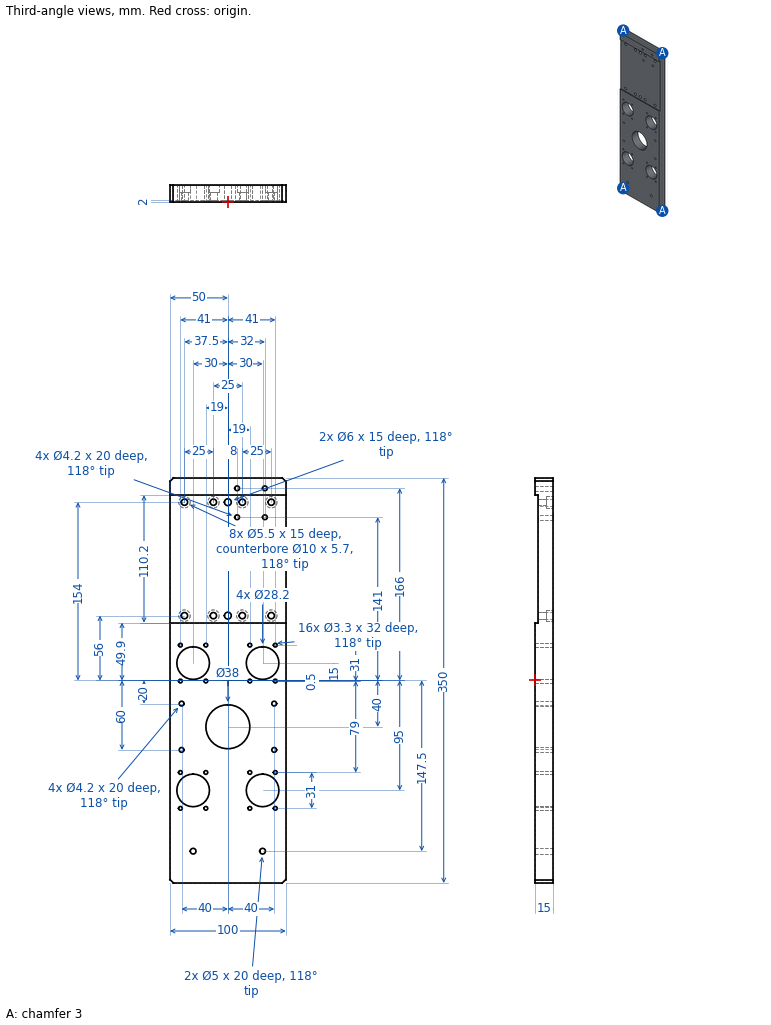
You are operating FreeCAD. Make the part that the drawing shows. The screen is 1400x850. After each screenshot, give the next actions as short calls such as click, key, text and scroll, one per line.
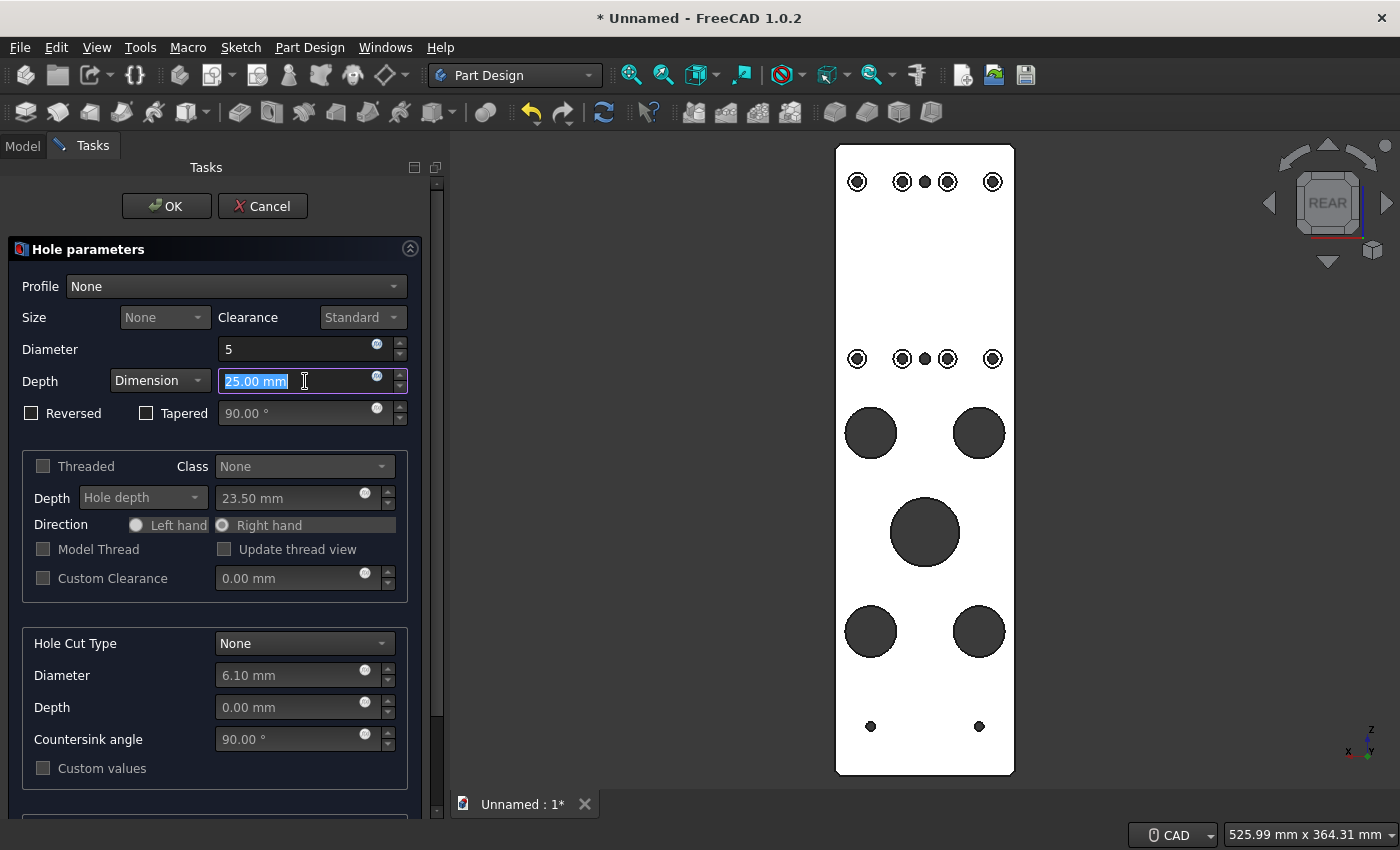
text(20)
key(Tab)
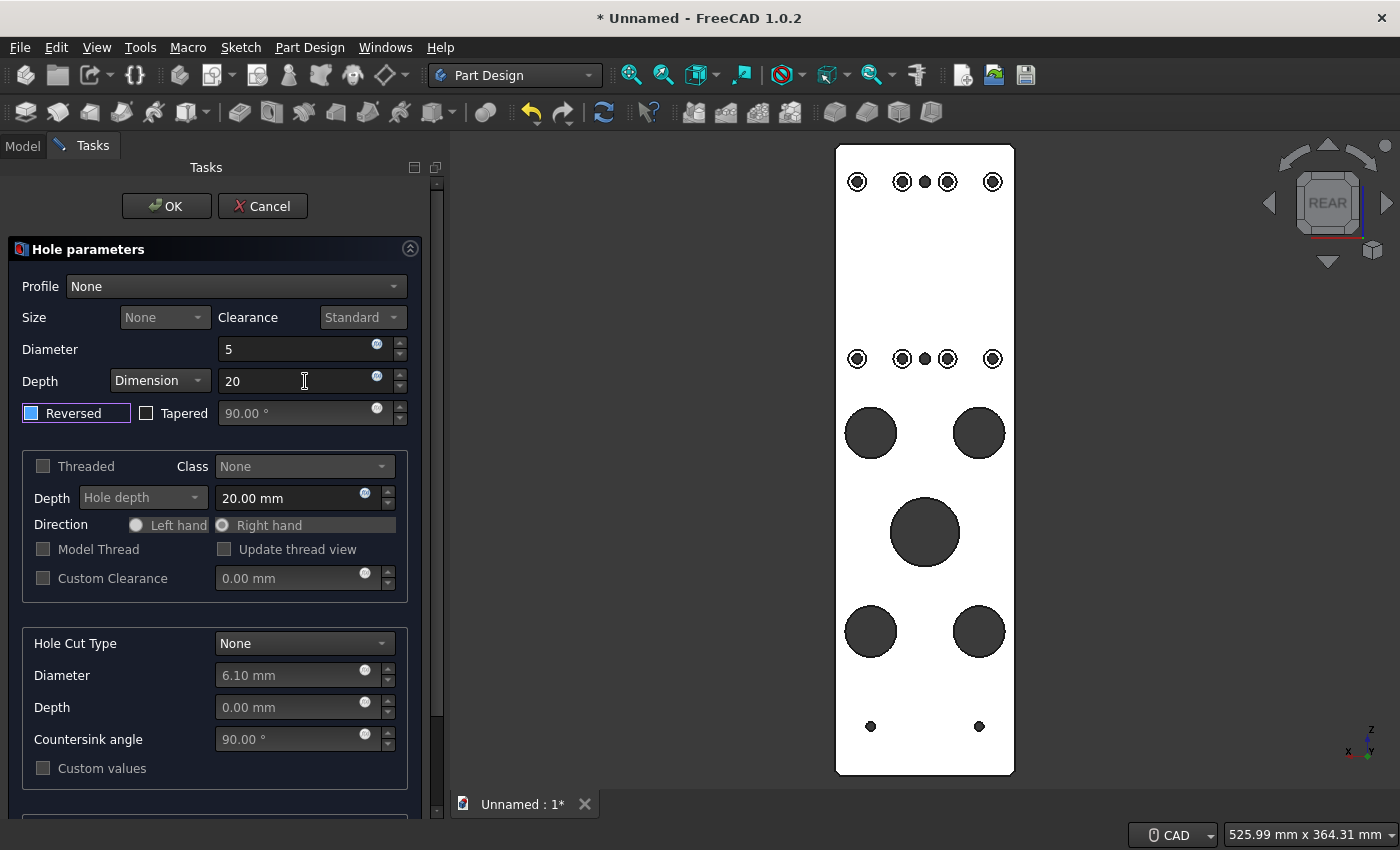
click(167, 206)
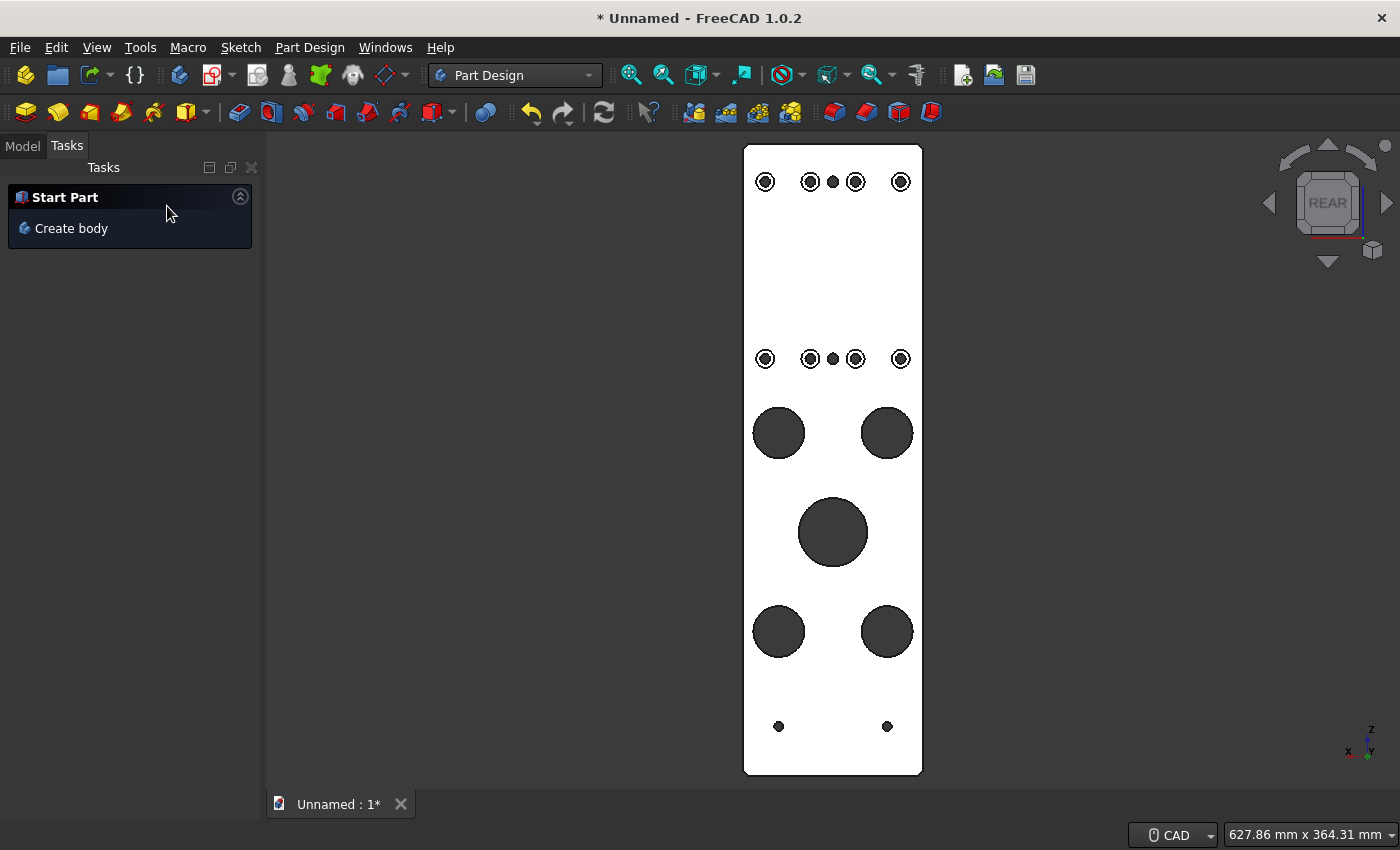
click(212, 76)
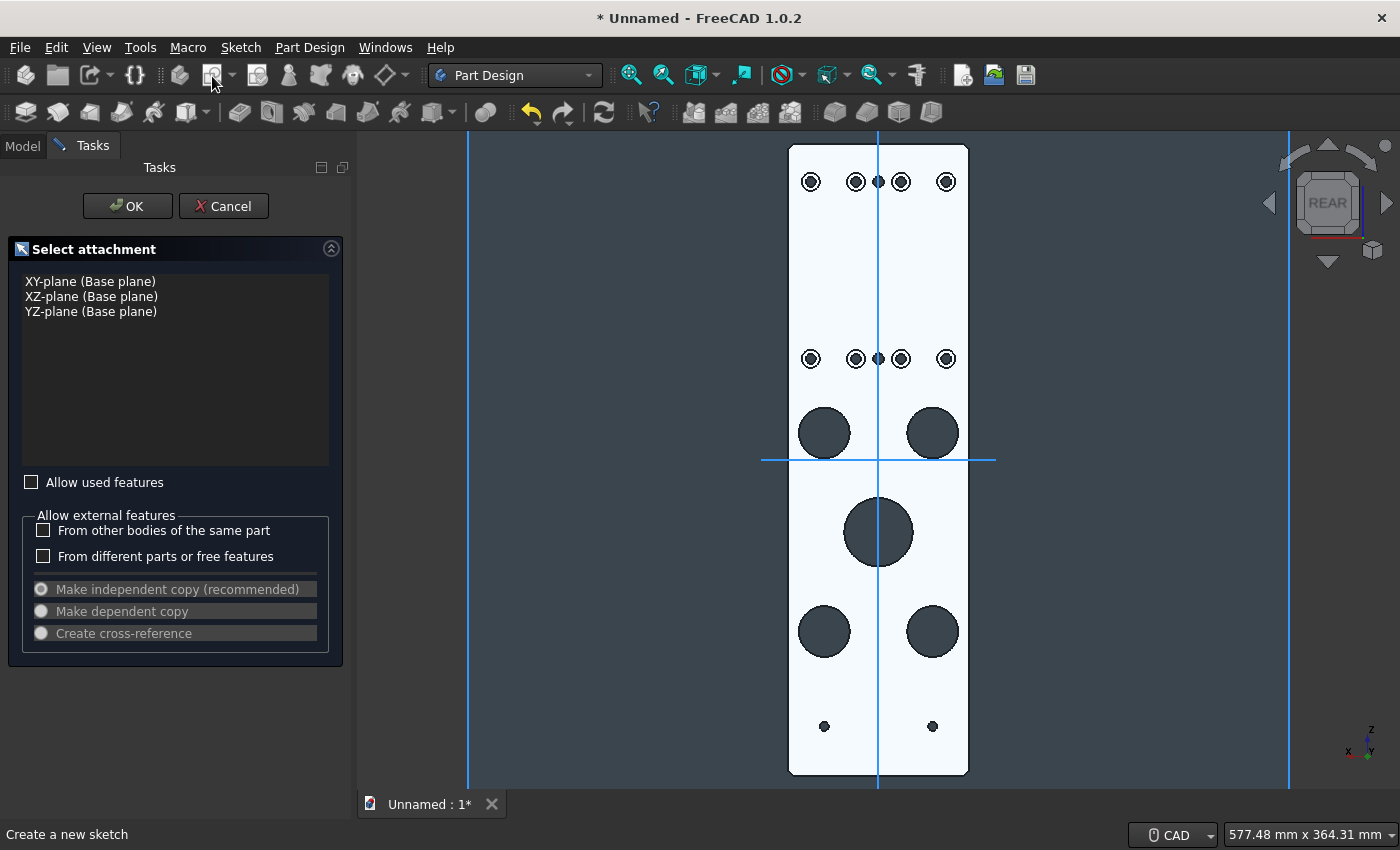
click(82, 296)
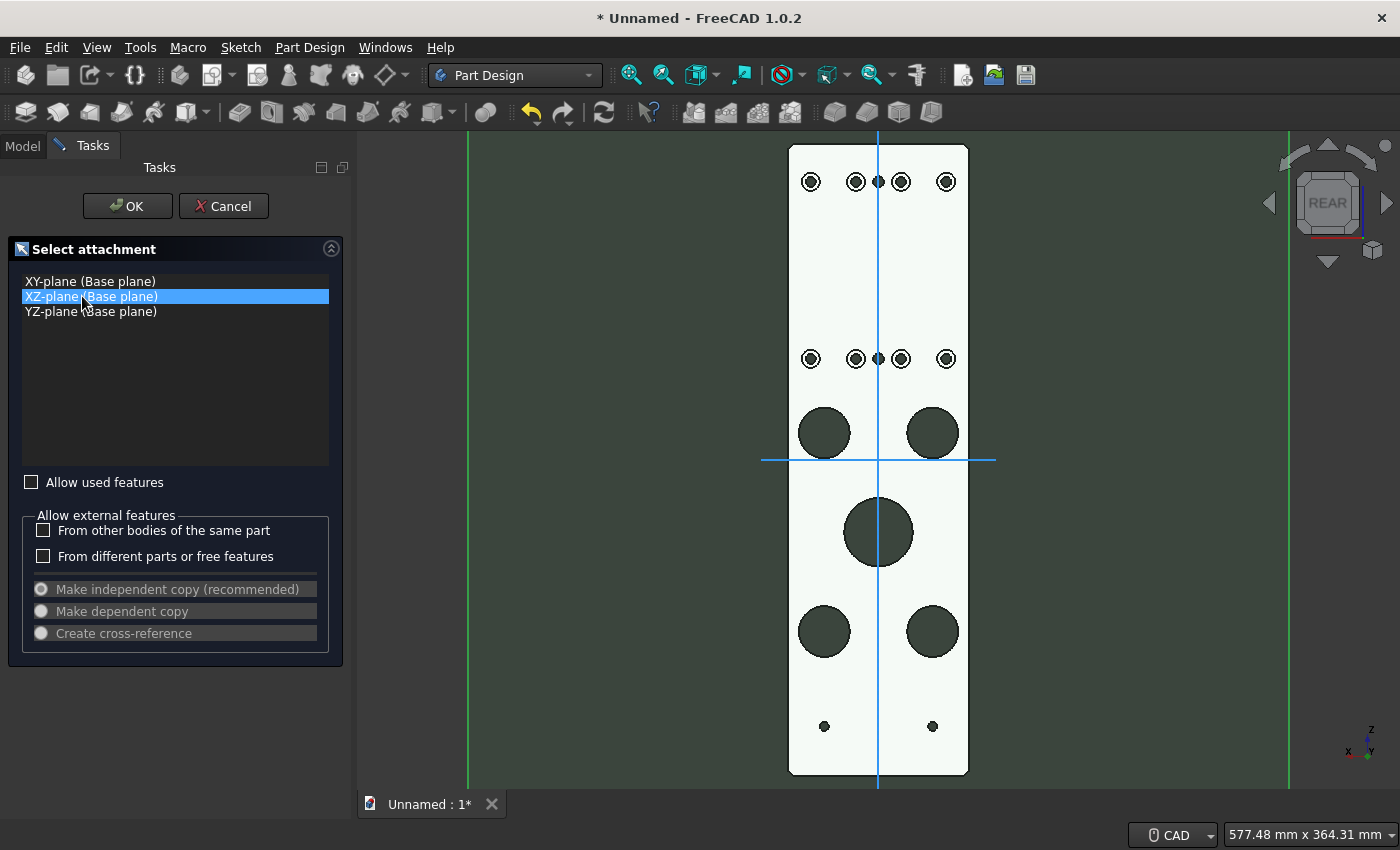
click(128, 206)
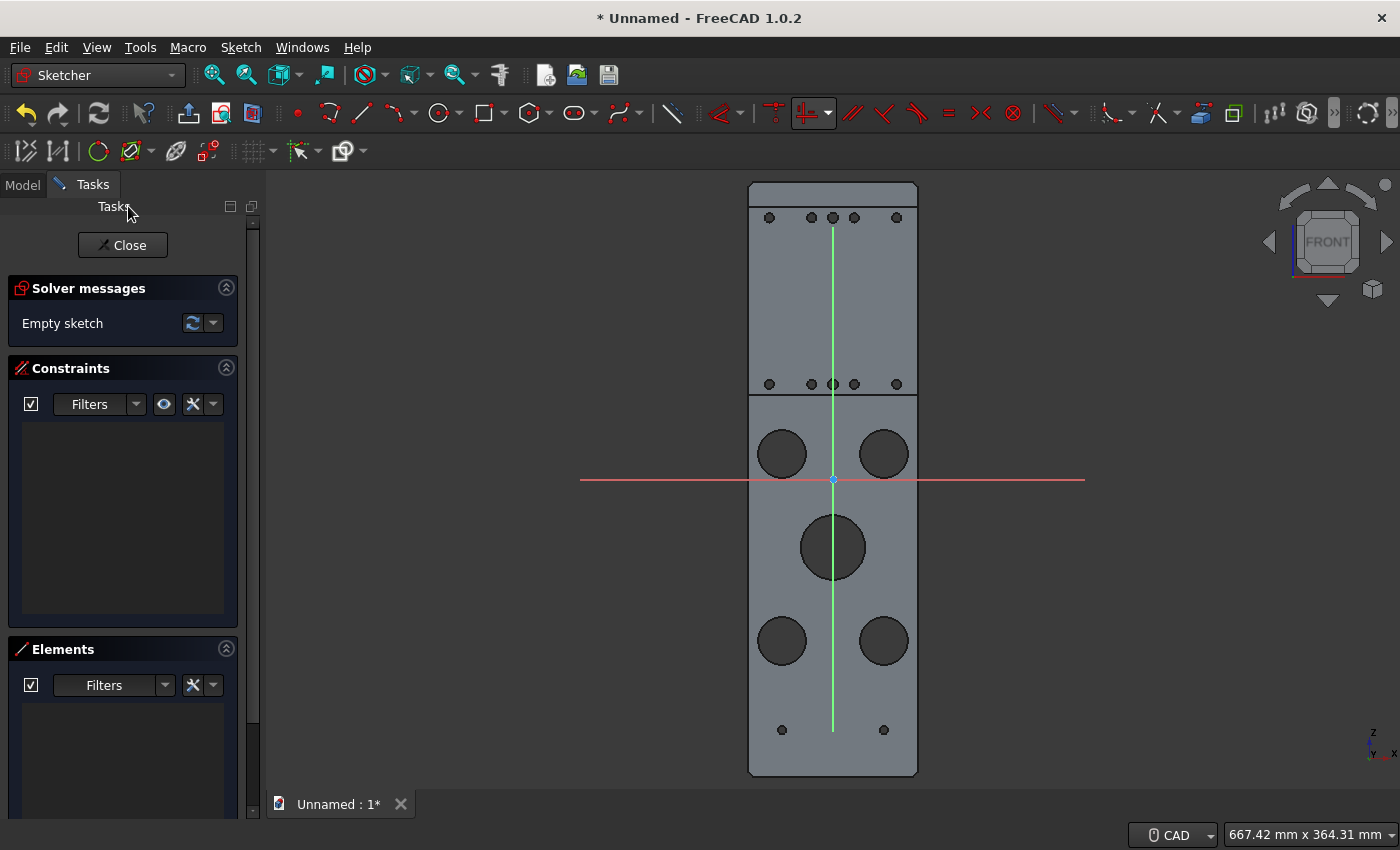
scroll(855, 550, up, 7)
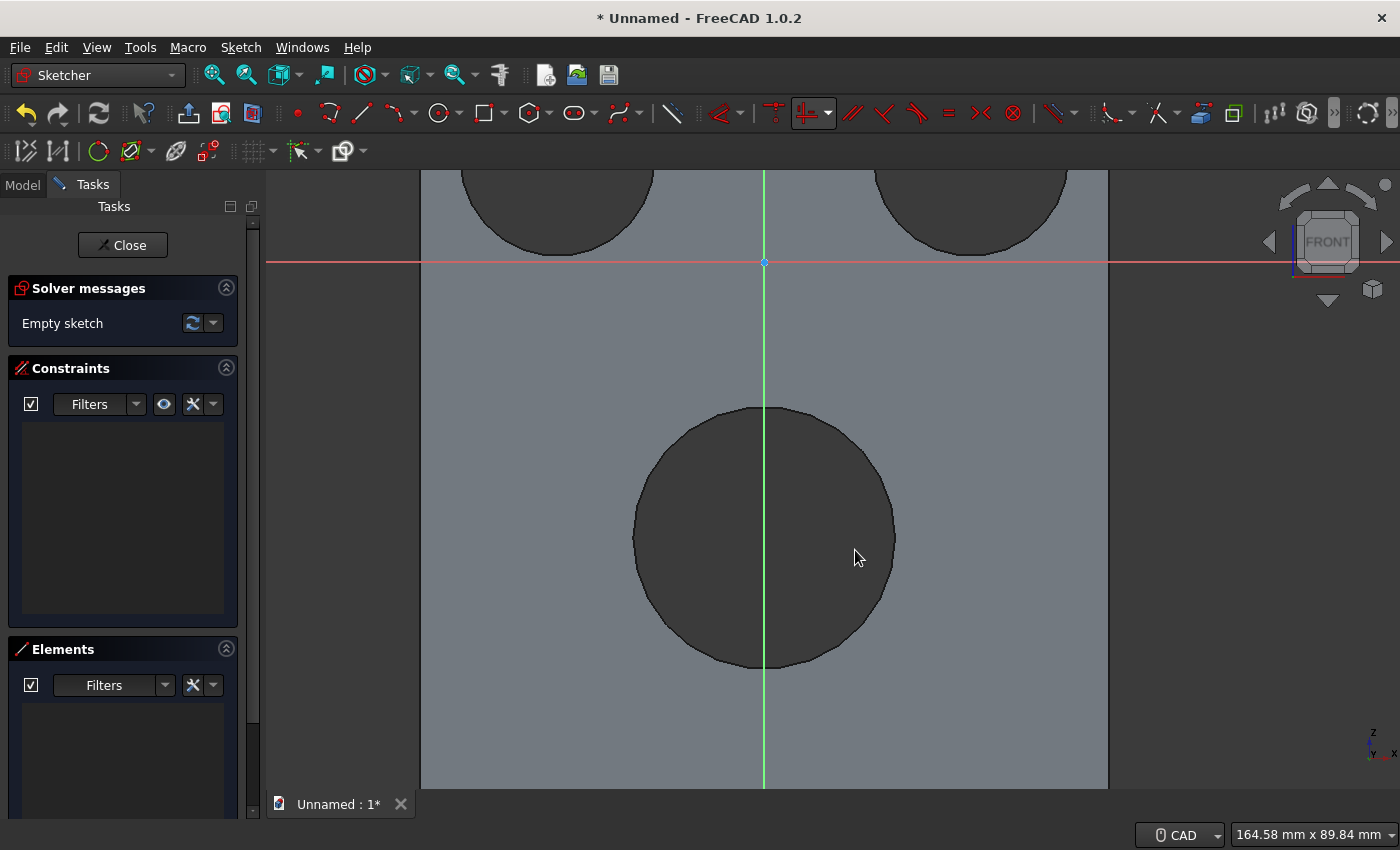
key(g)
key(c)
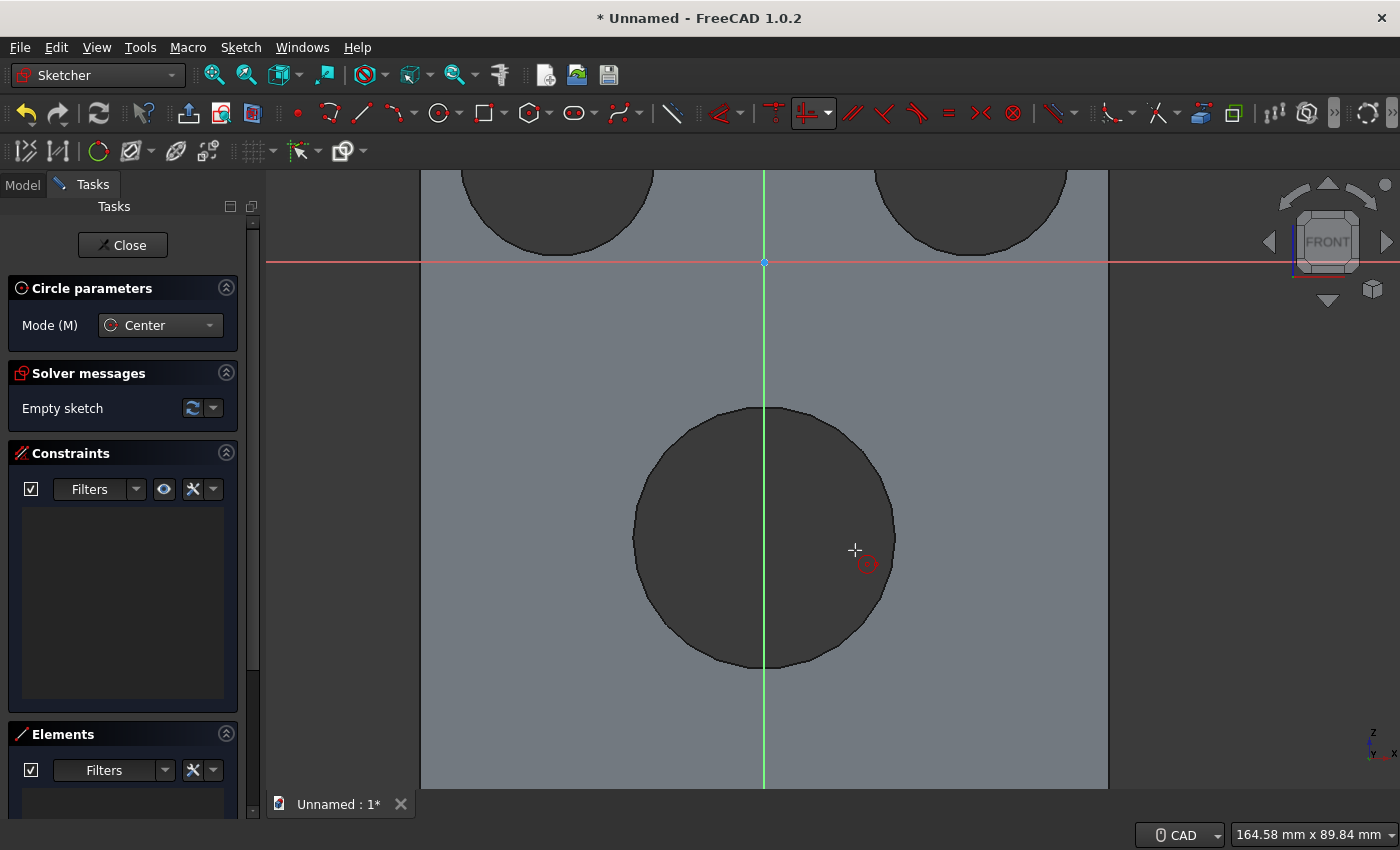
scroll(489, 400, up, 3)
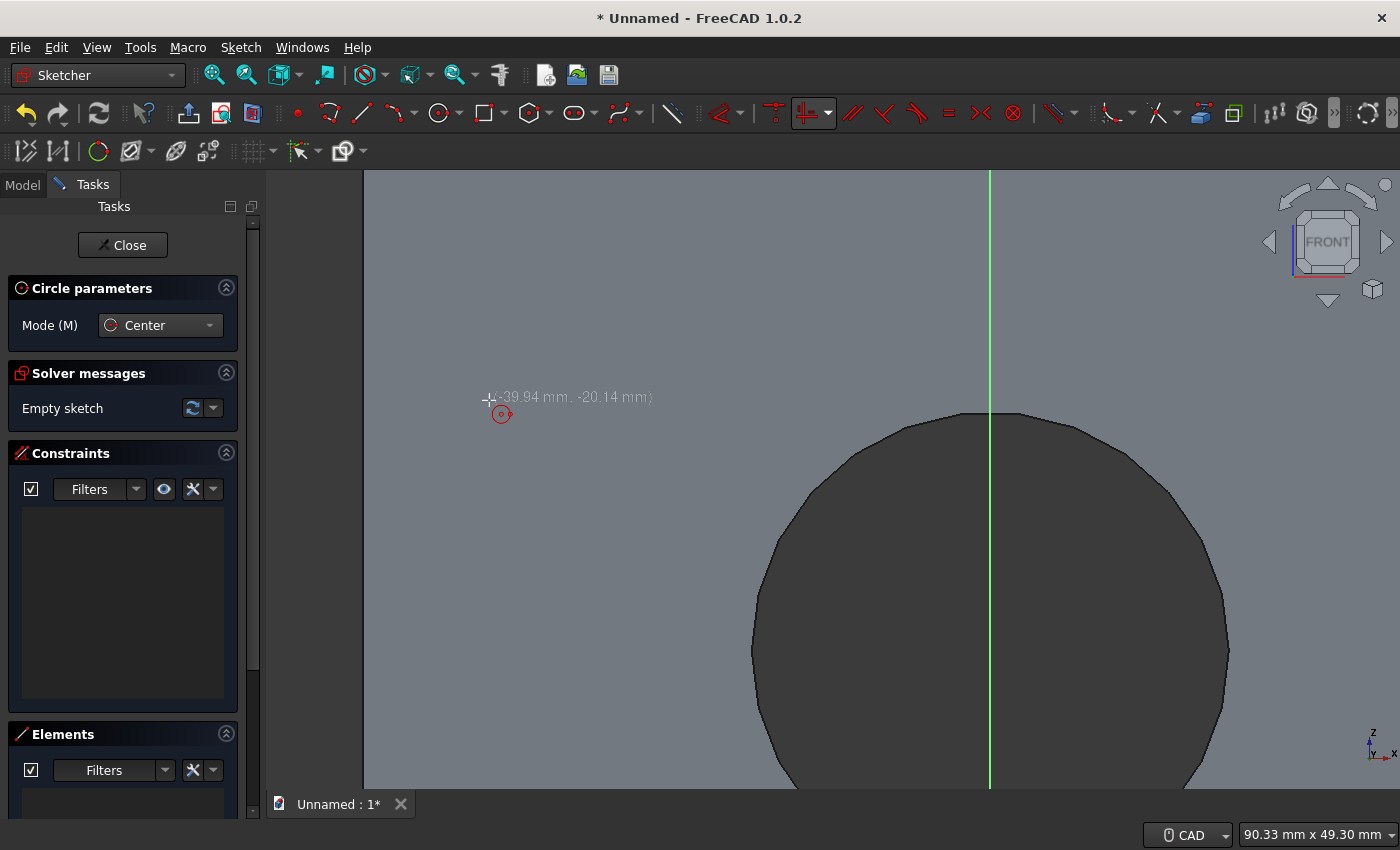
click(488, 400)
click(507, 381)